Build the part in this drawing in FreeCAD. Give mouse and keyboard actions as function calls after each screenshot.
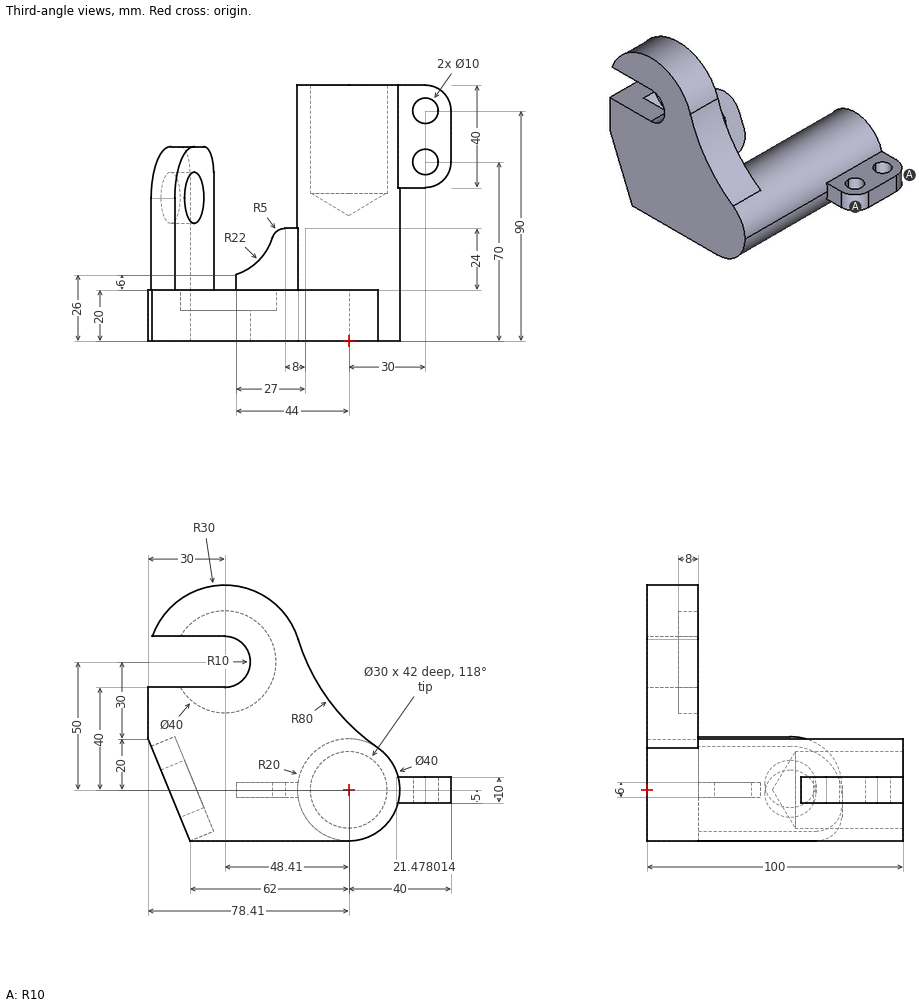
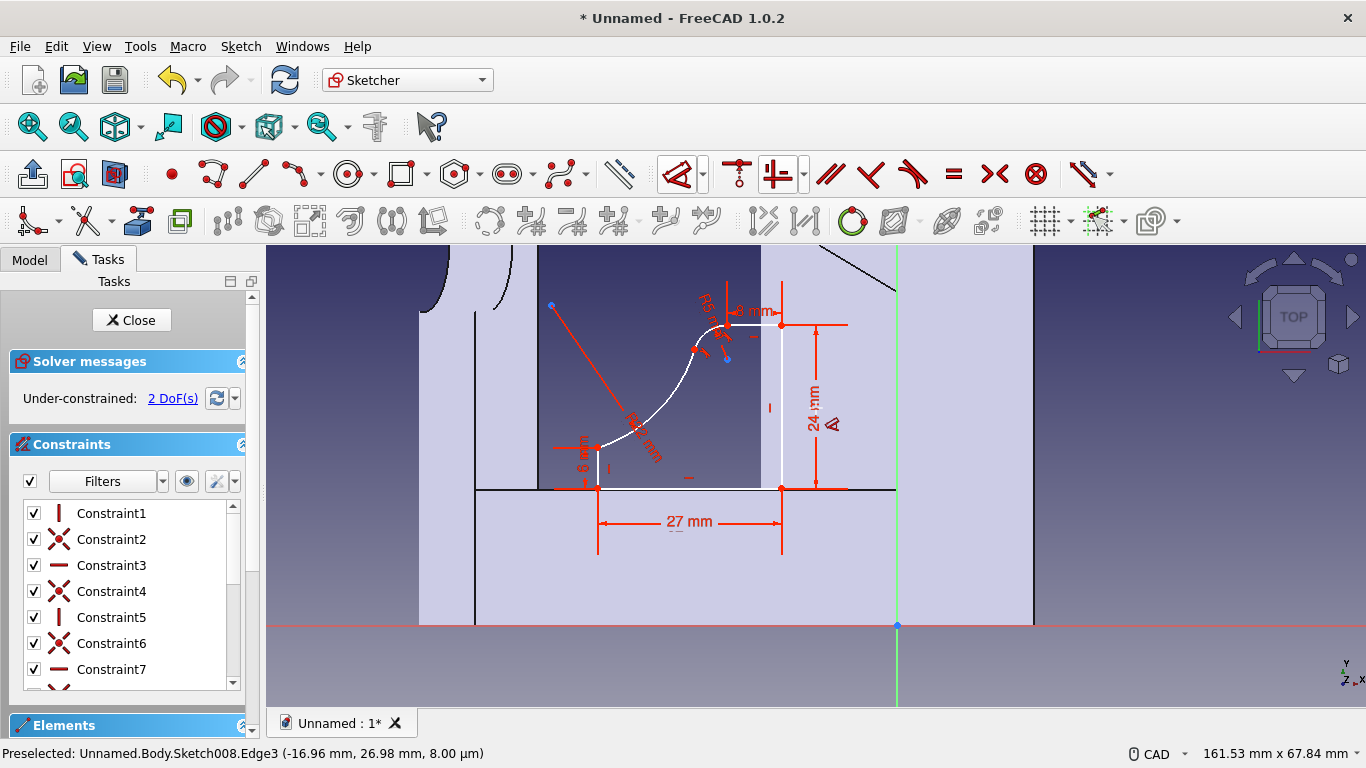
click(598, 448)
click(748, 660)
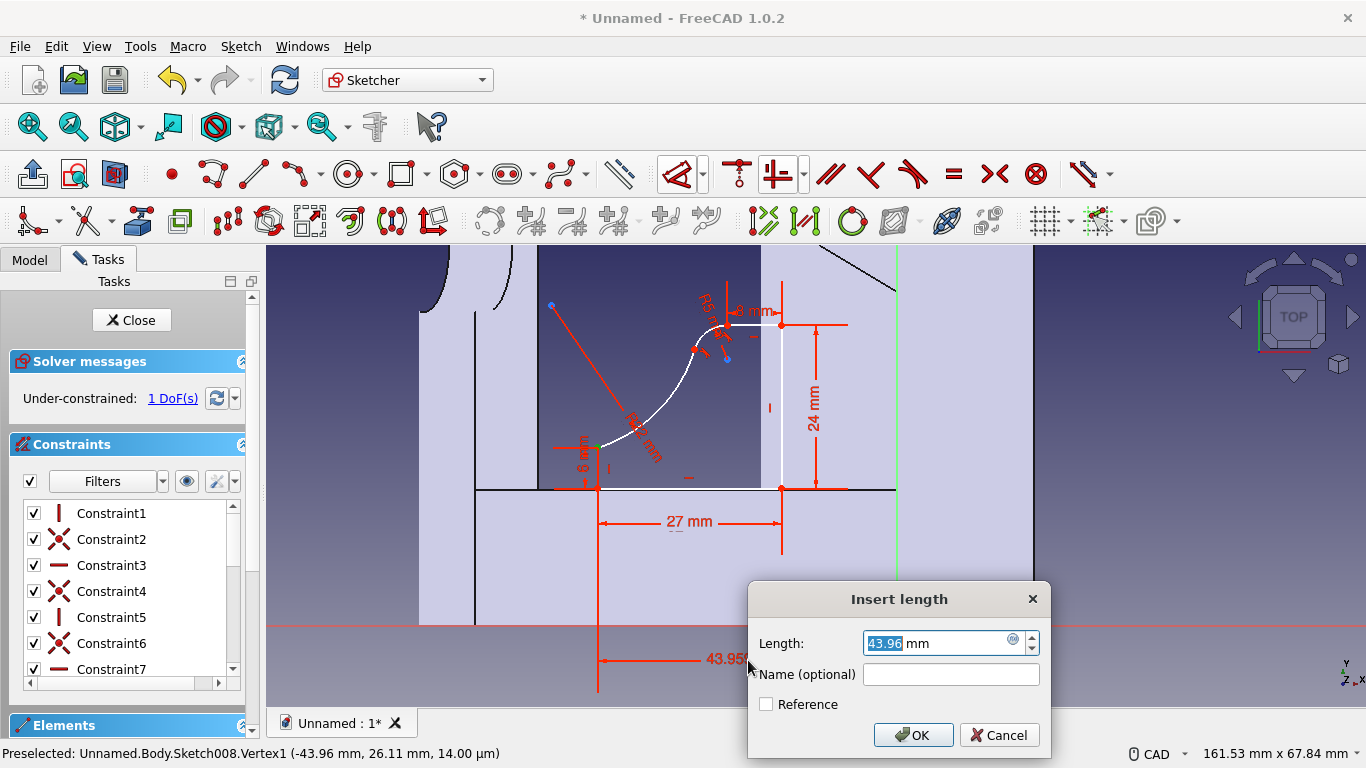
text(44)
key(Return)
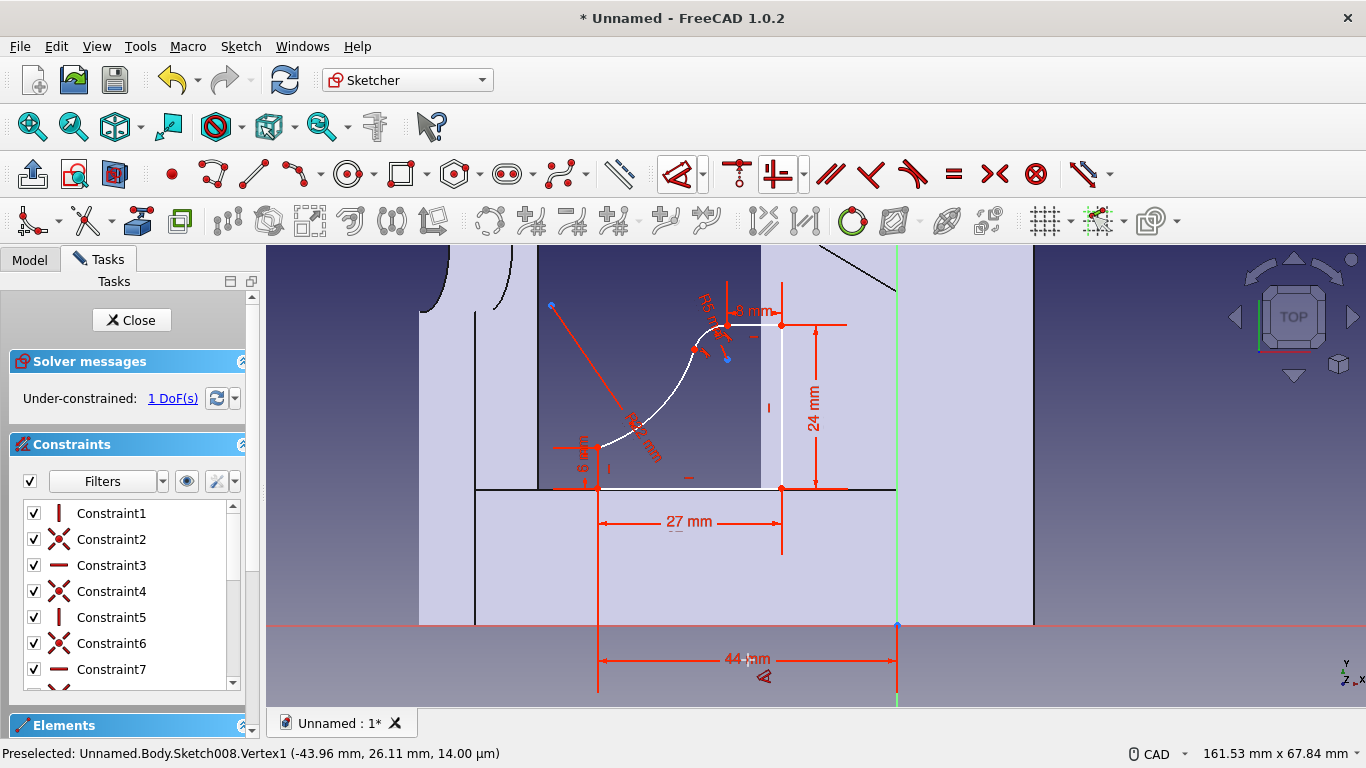
click(598, 448)
click(931, 537)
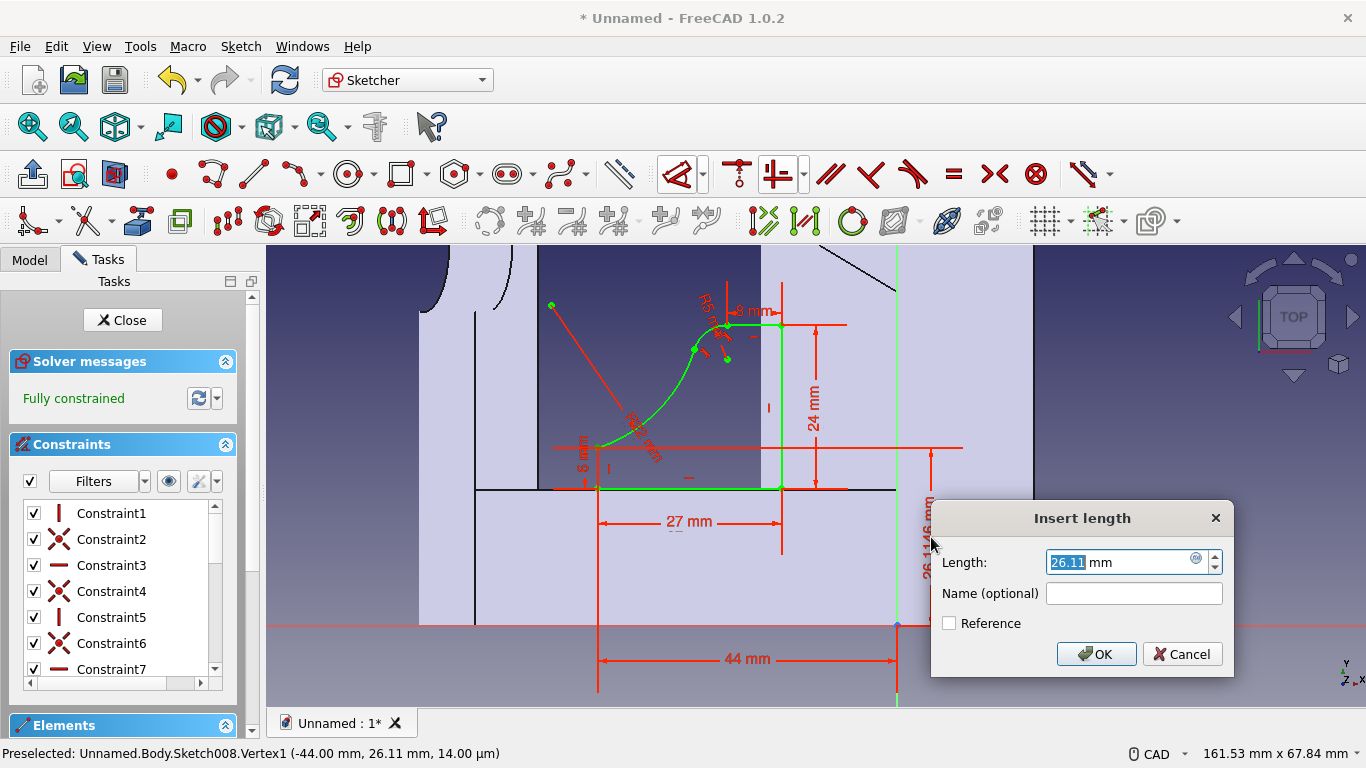
text(26)
key(Return)
key(Escape)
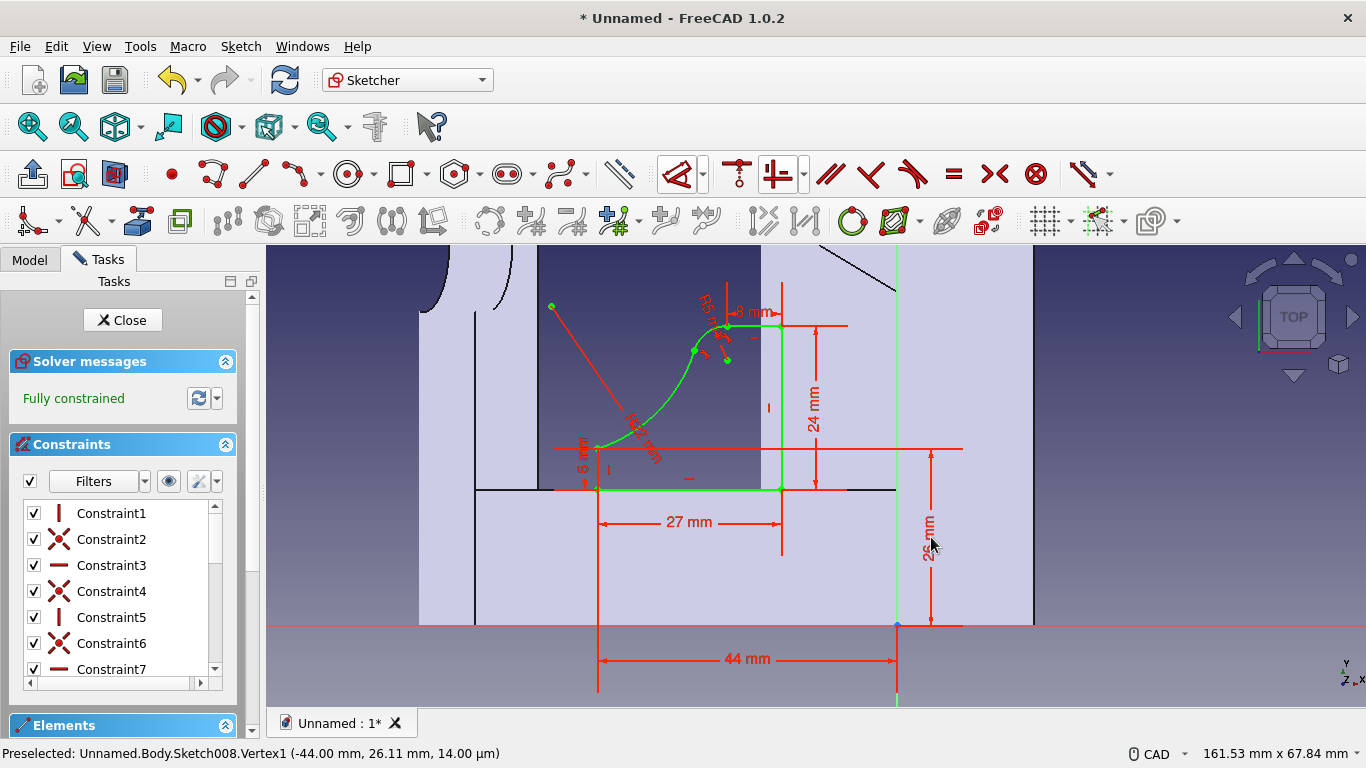
click(123, 320)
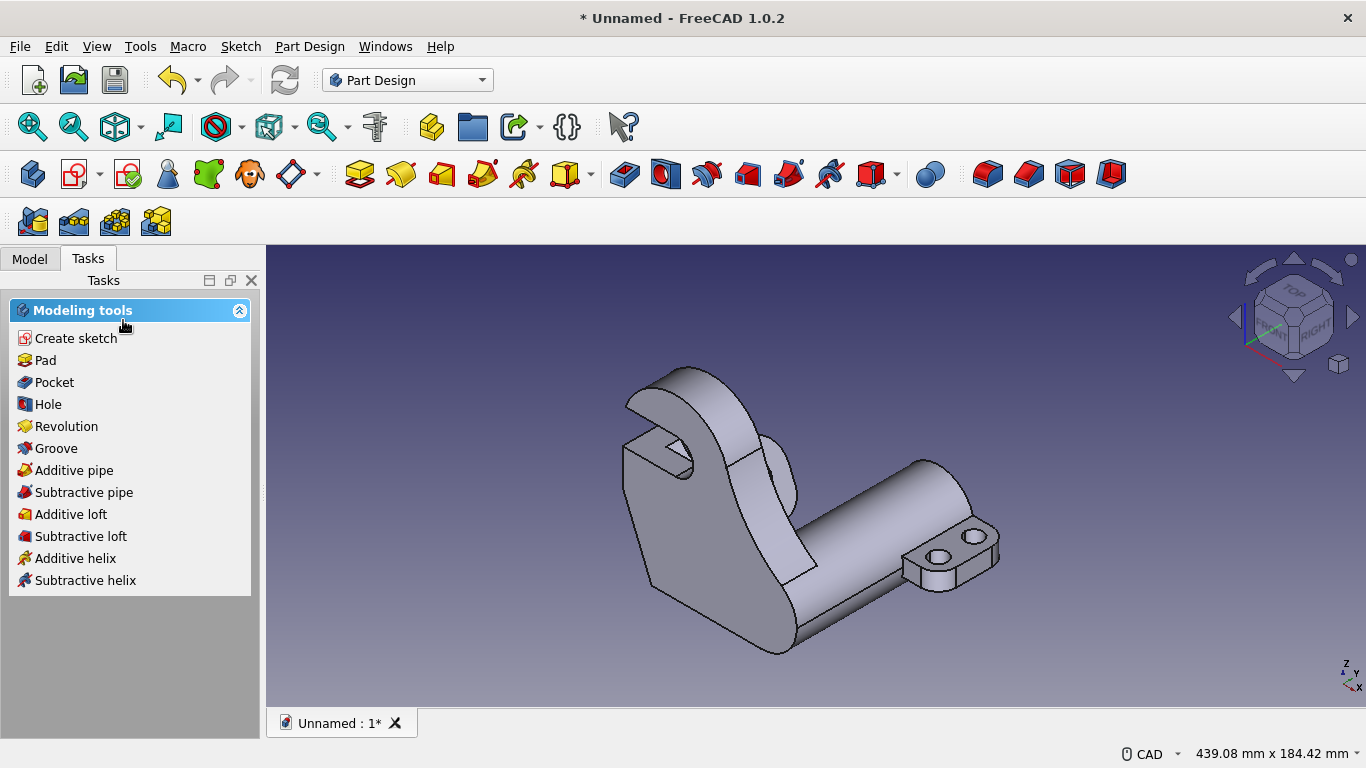
click(360, 174)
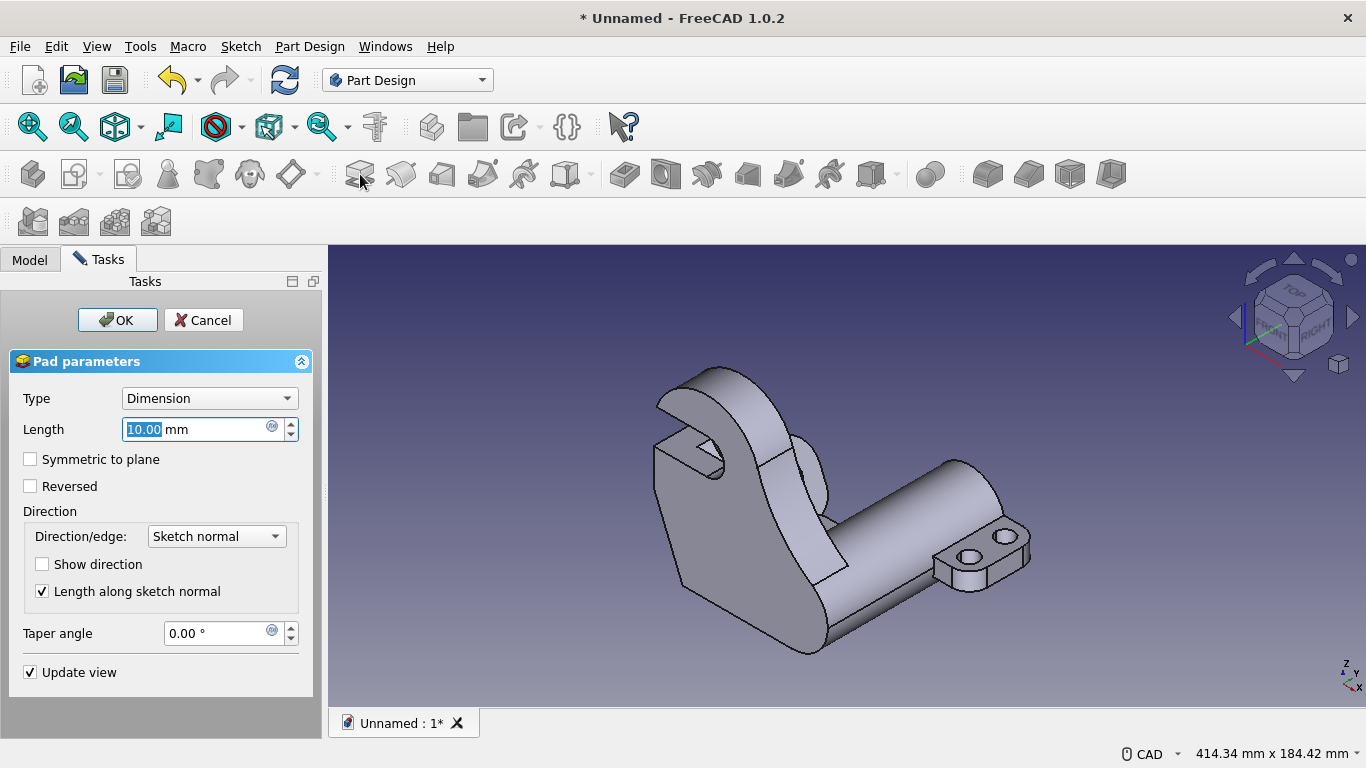
text(6)
key(Tab)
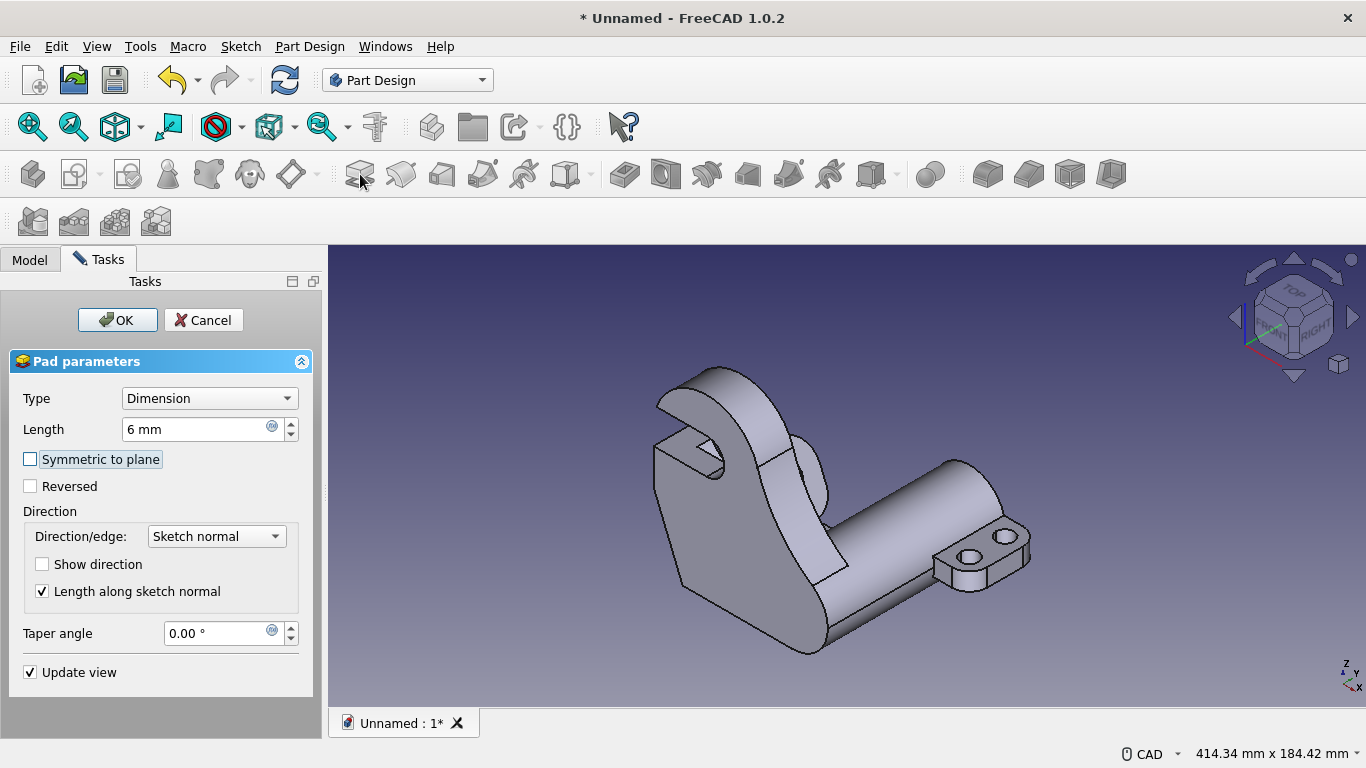
click(31, 459)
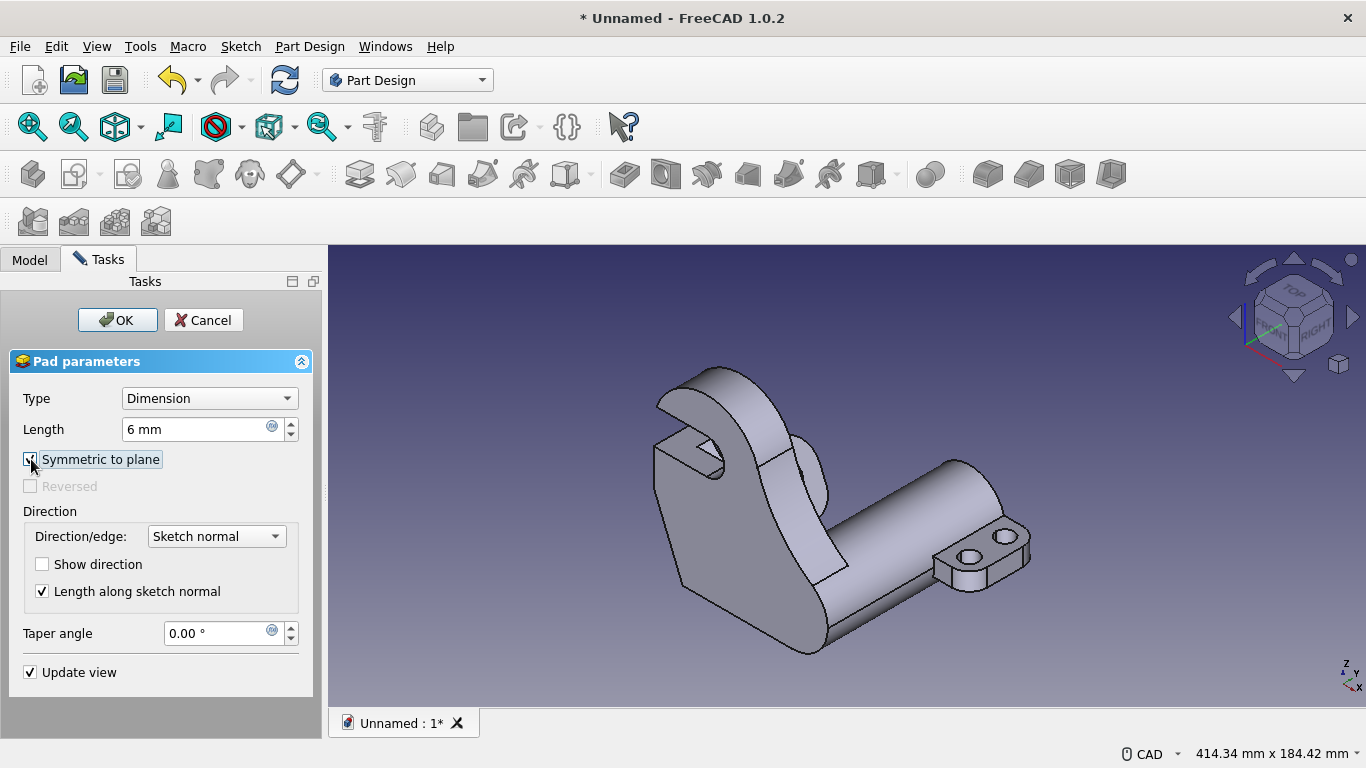
click(118, 320)